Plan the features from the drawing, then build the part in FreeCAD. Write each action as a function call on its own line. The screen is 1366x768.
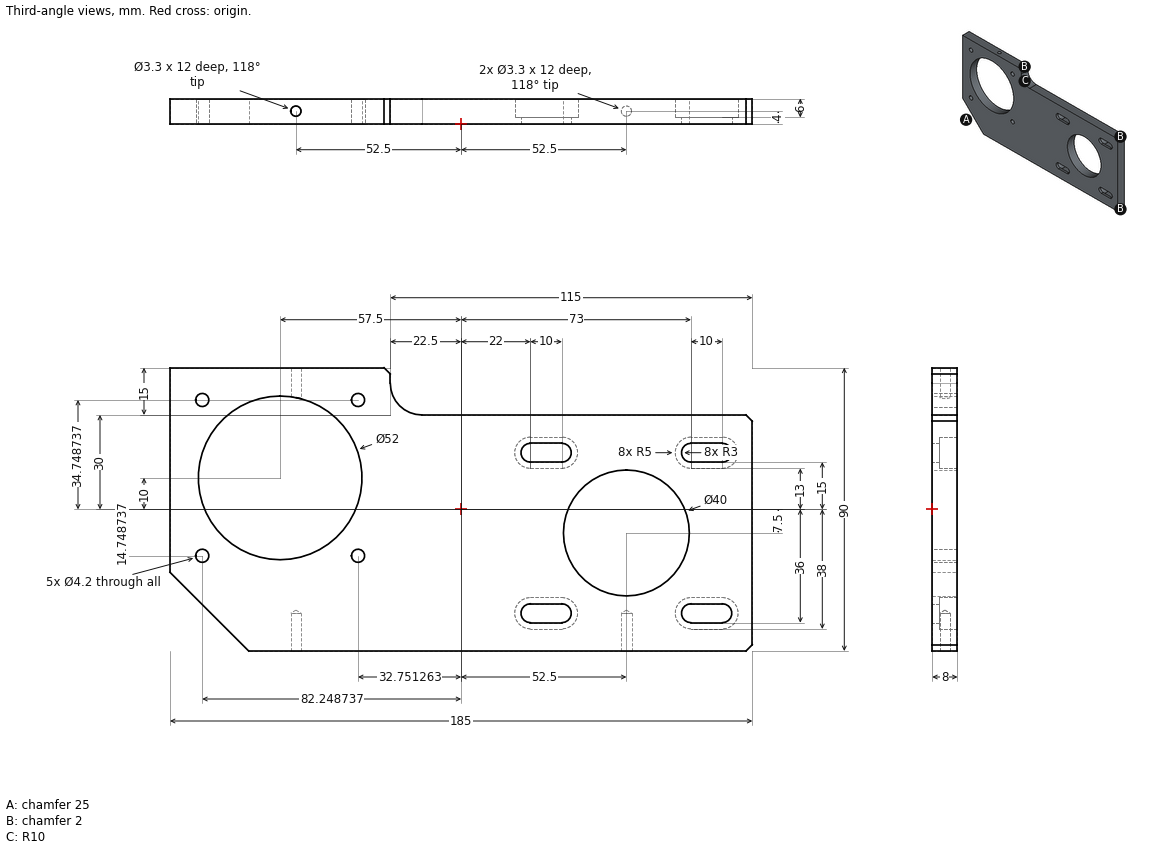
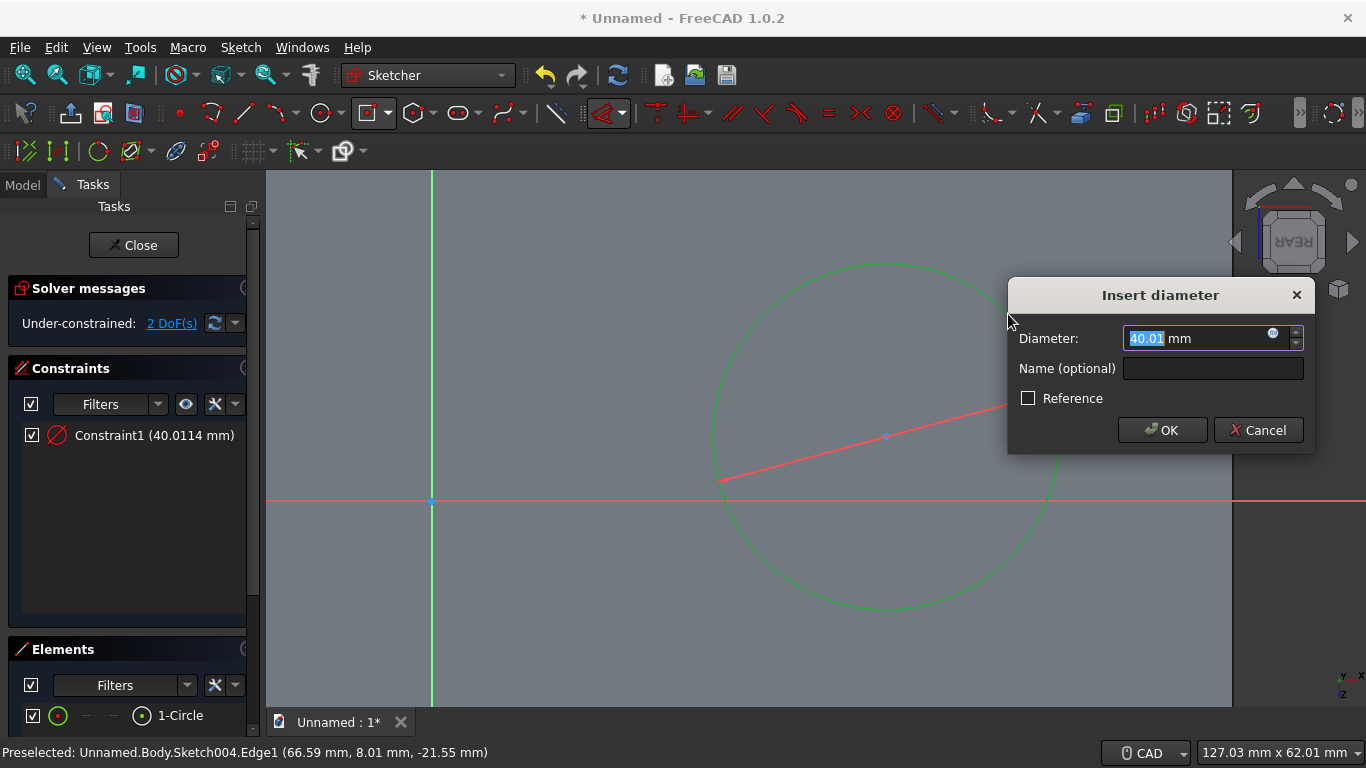
text(40)
key(Return)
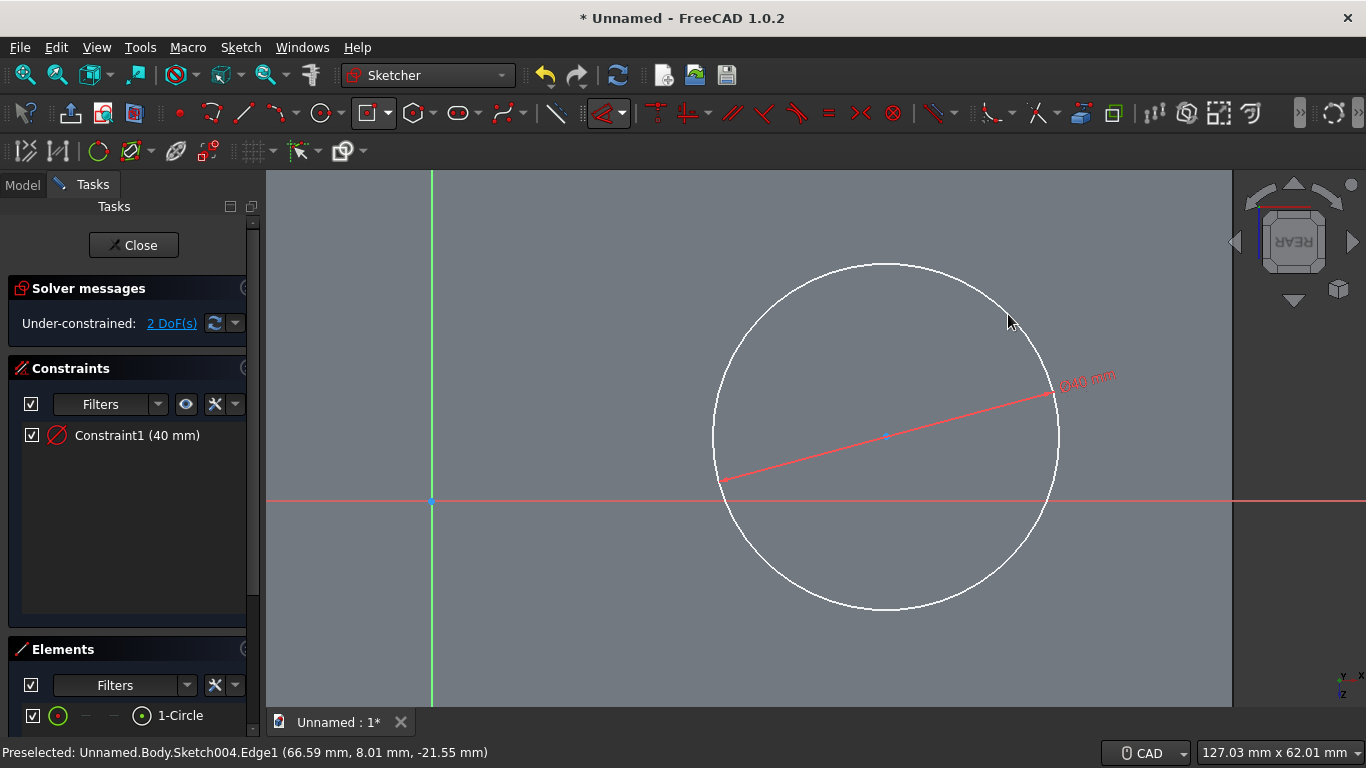
click(886, 437)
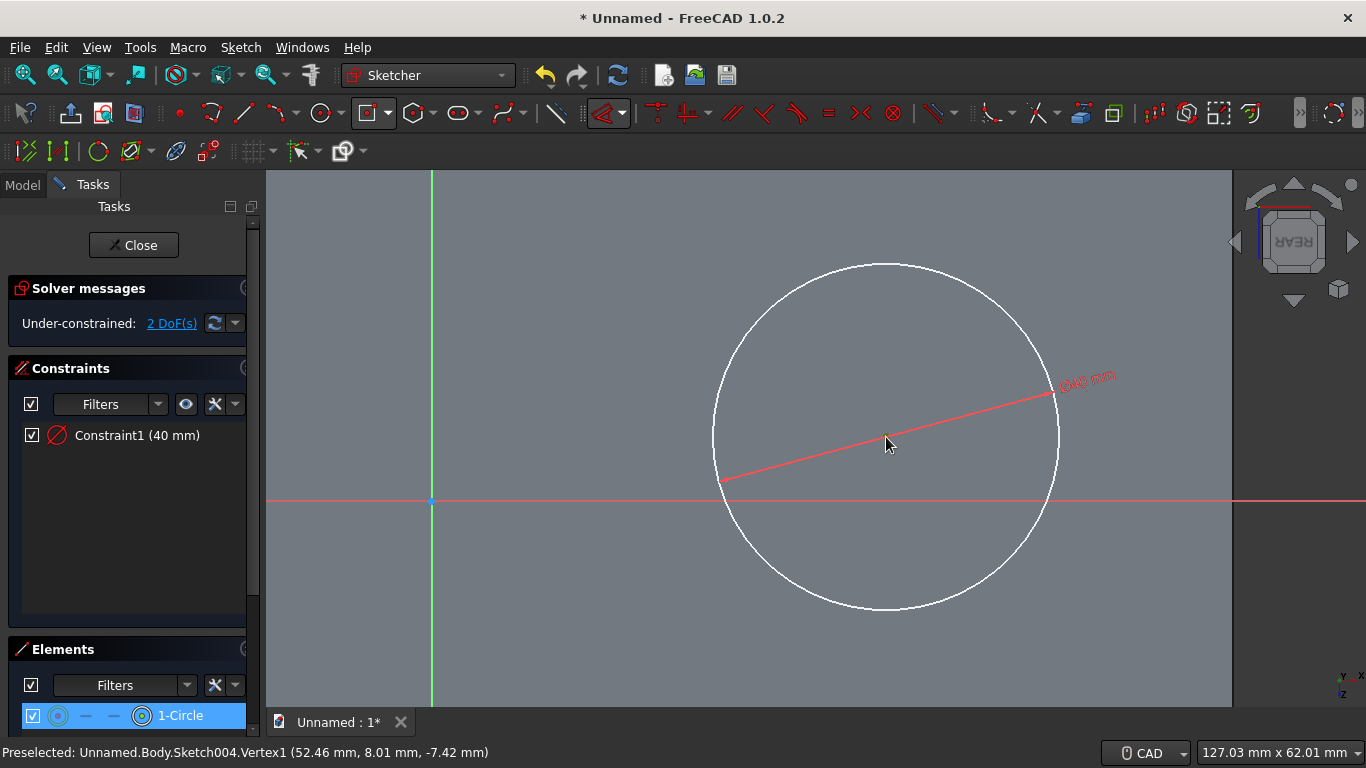
click(624, 114)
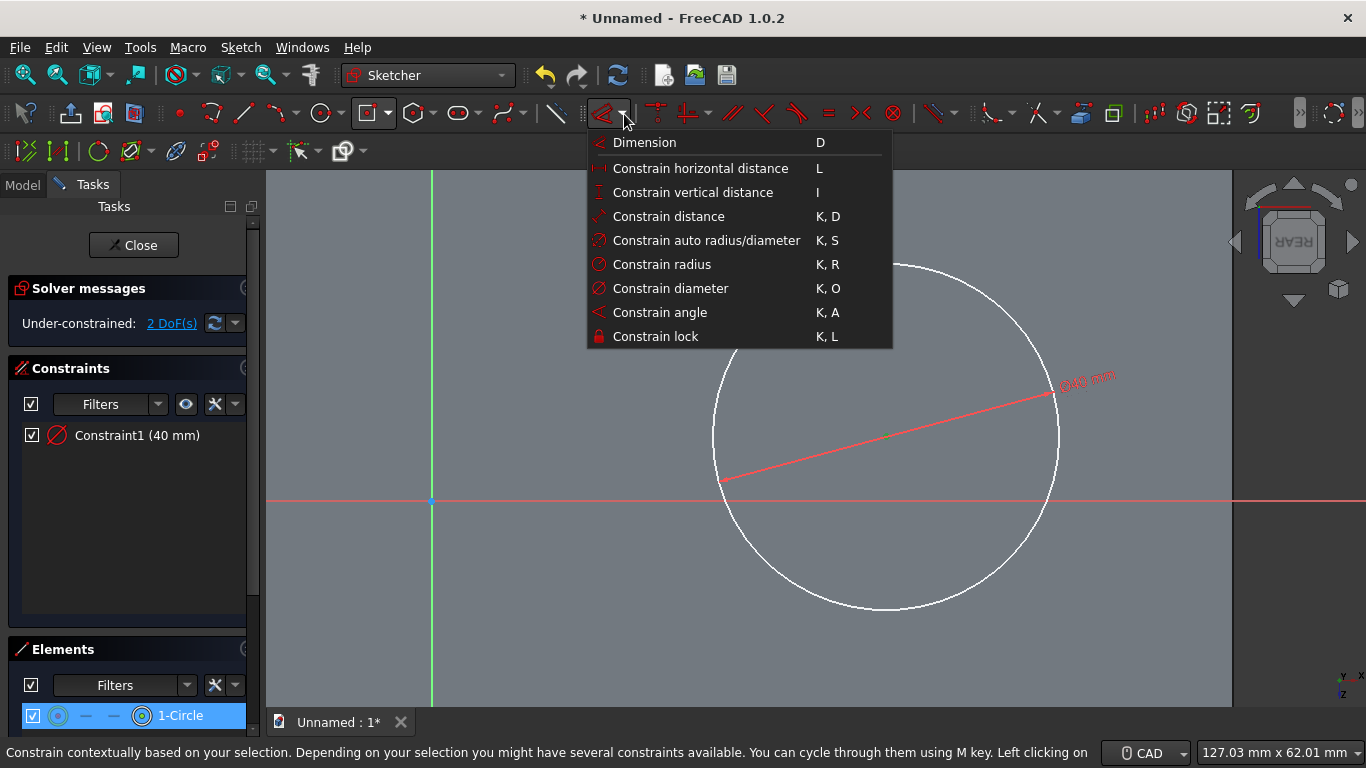
click(740, 192)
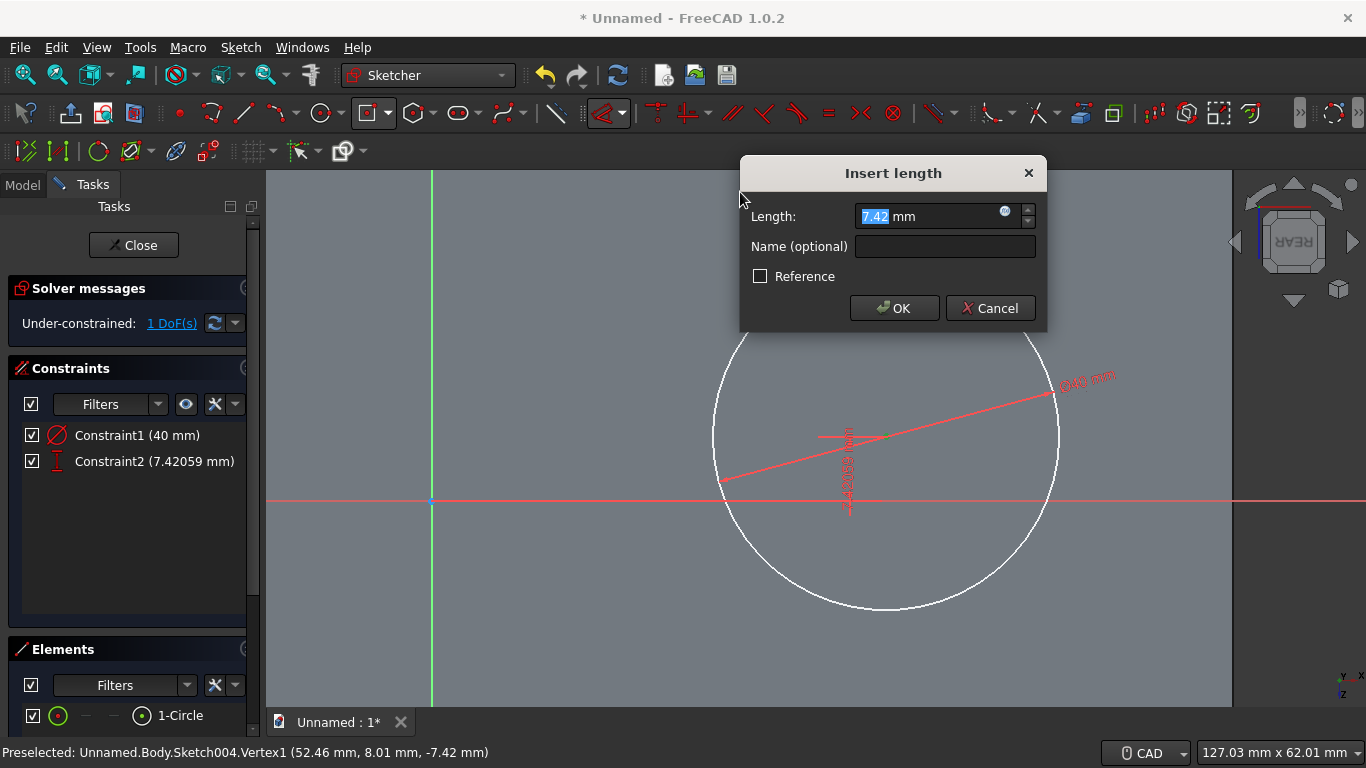
text(7.5)
key(Return)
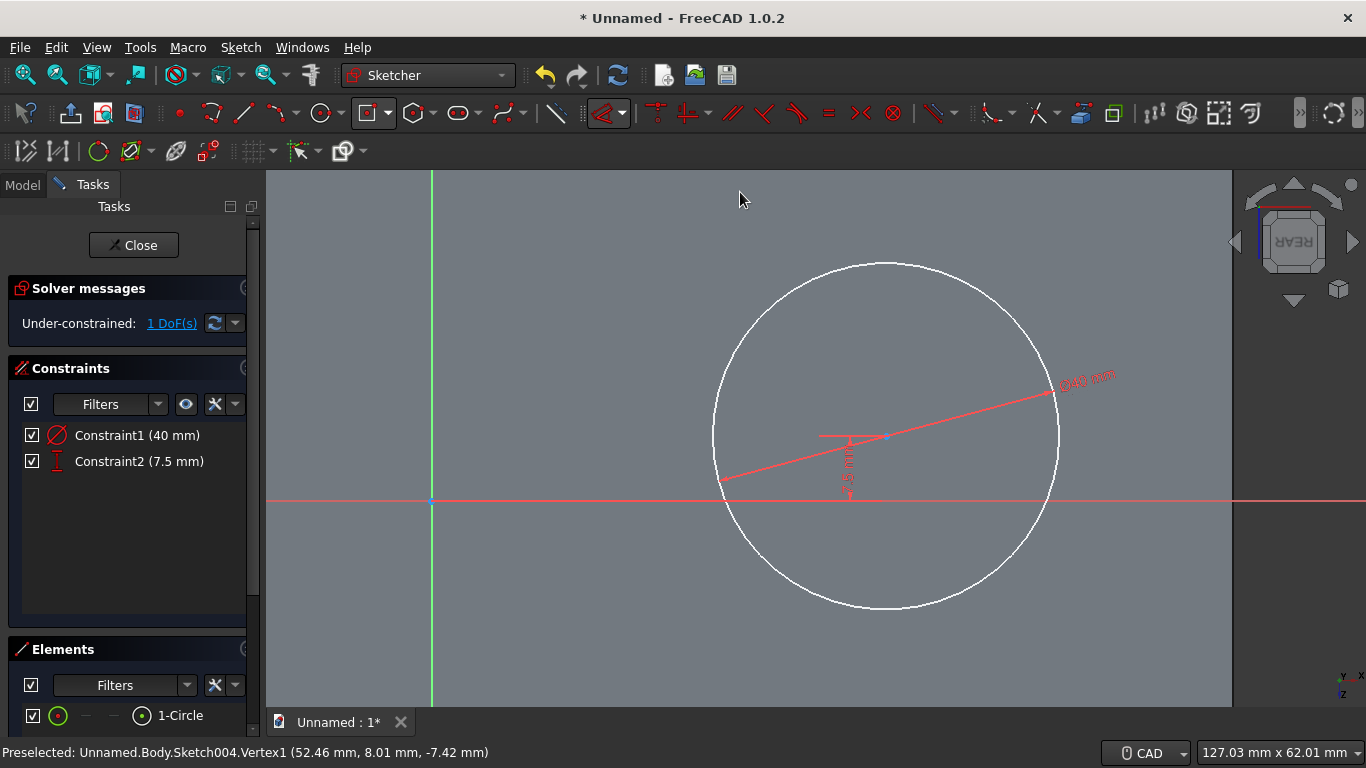
click(886, 436)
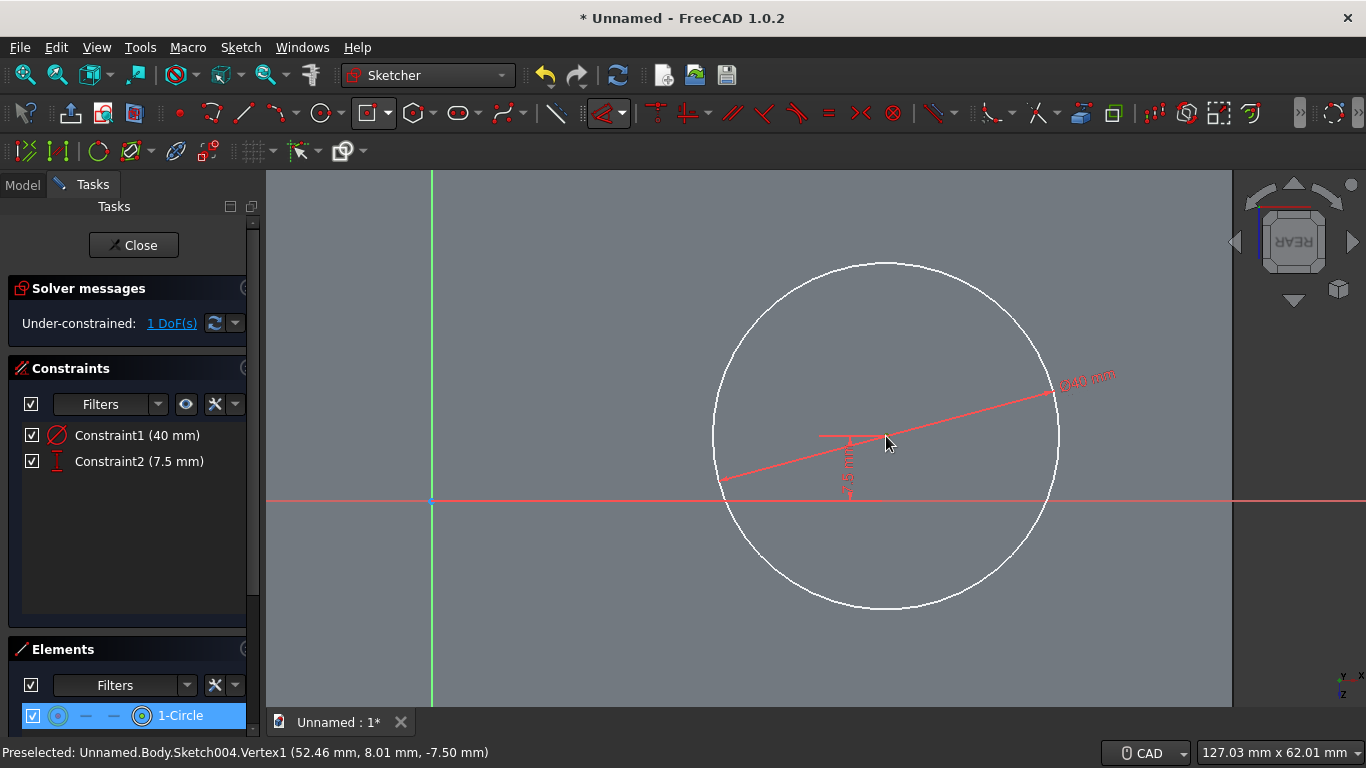
key(l)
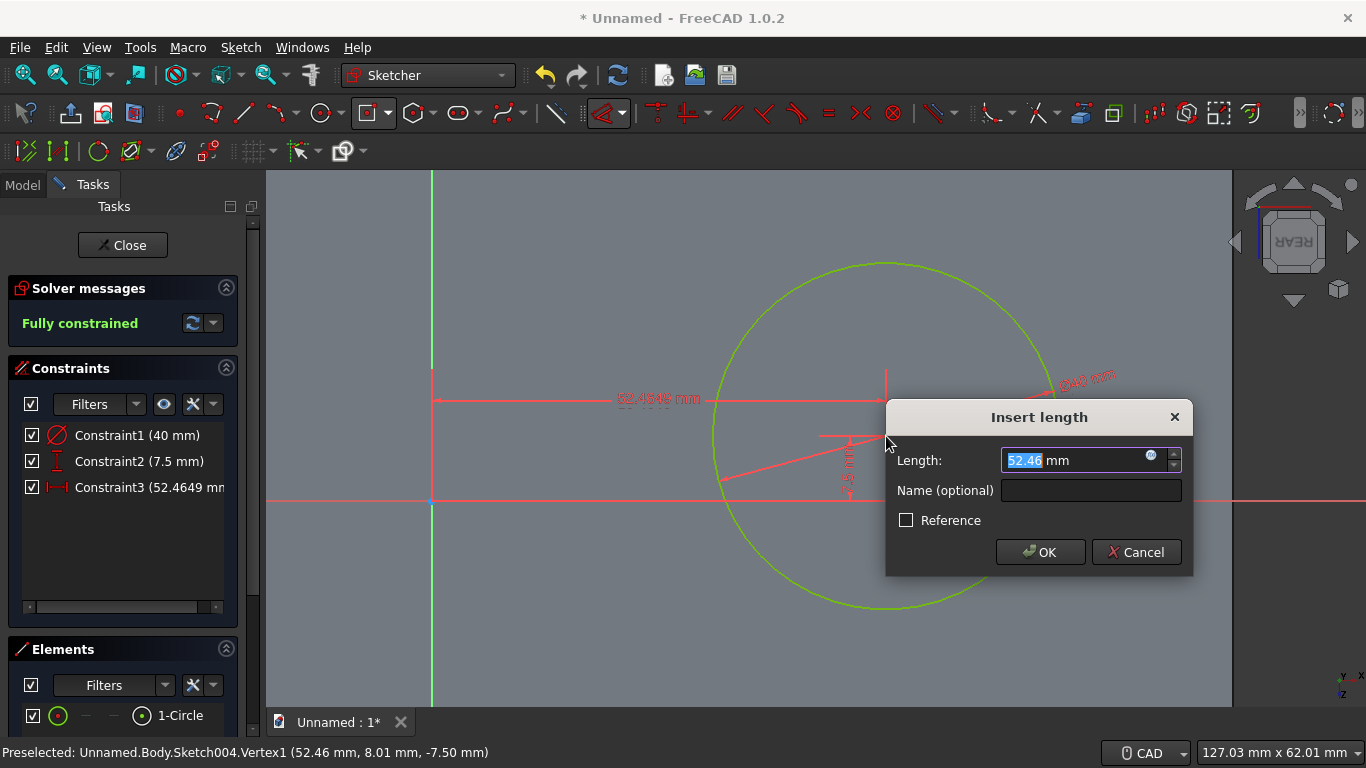
text(52.5)
key(Return)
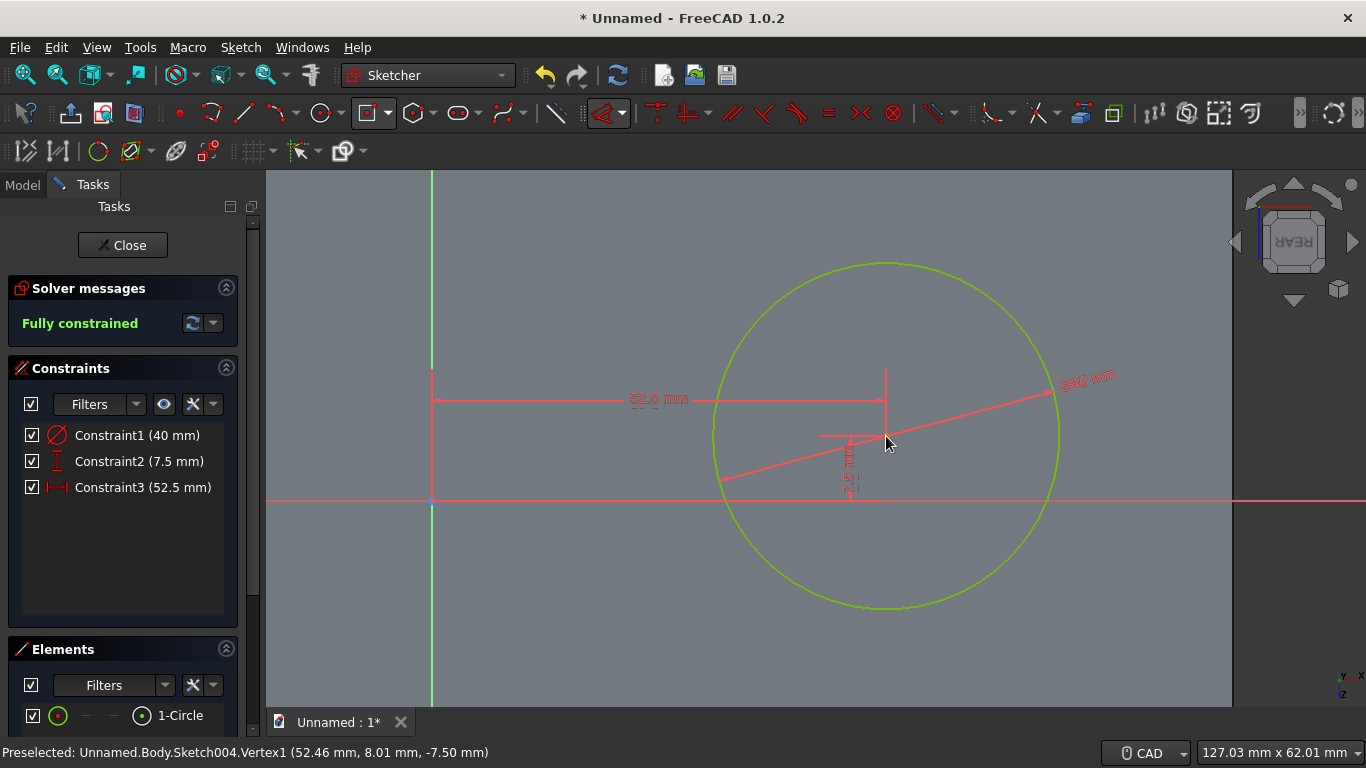
click(123, 245)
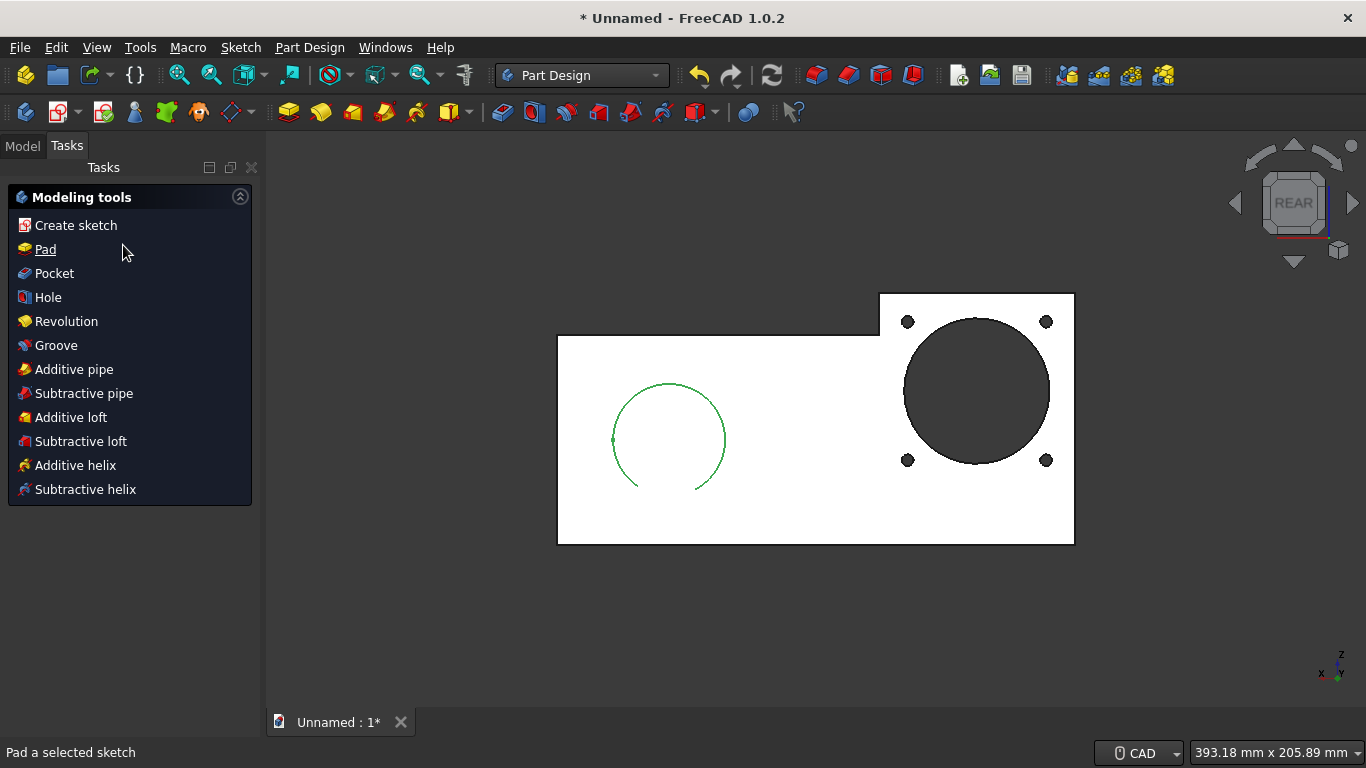
click(504, 112)